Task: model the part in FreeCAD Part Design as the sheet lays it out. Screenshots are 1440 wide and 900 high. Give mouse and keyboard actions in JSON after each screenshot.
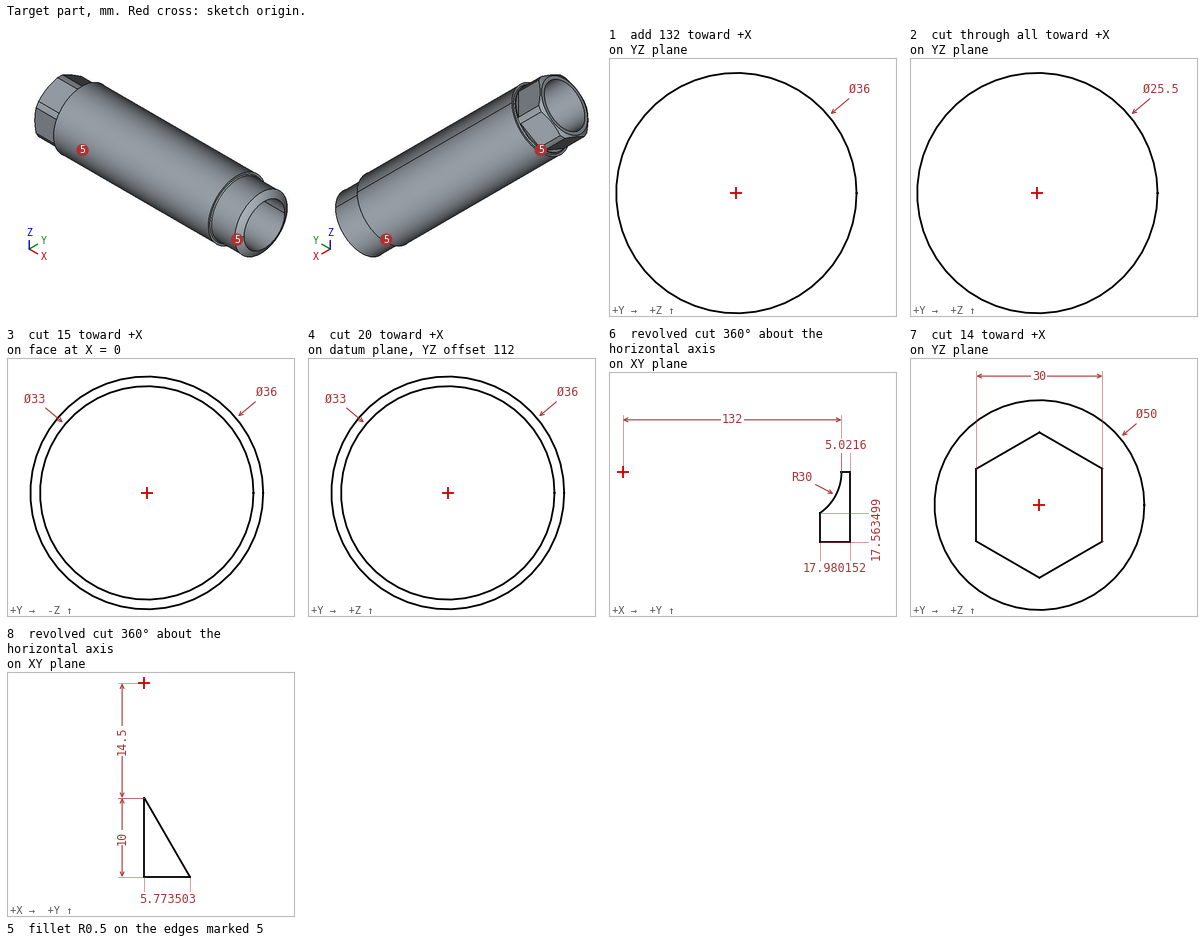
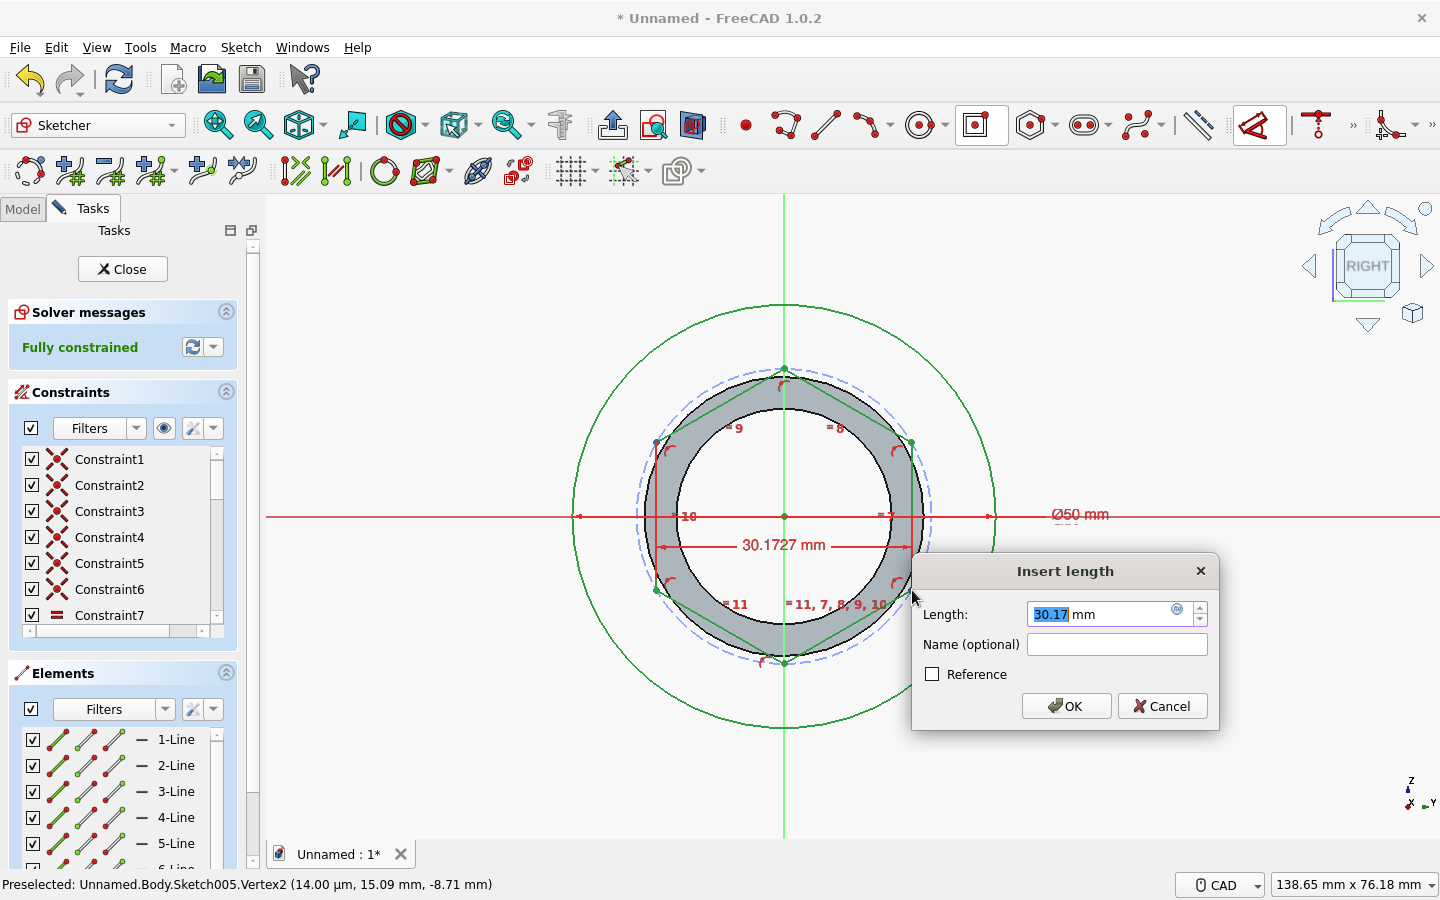
{"action": "type", "text": "30"}
{"action": "key", "text": "Return"}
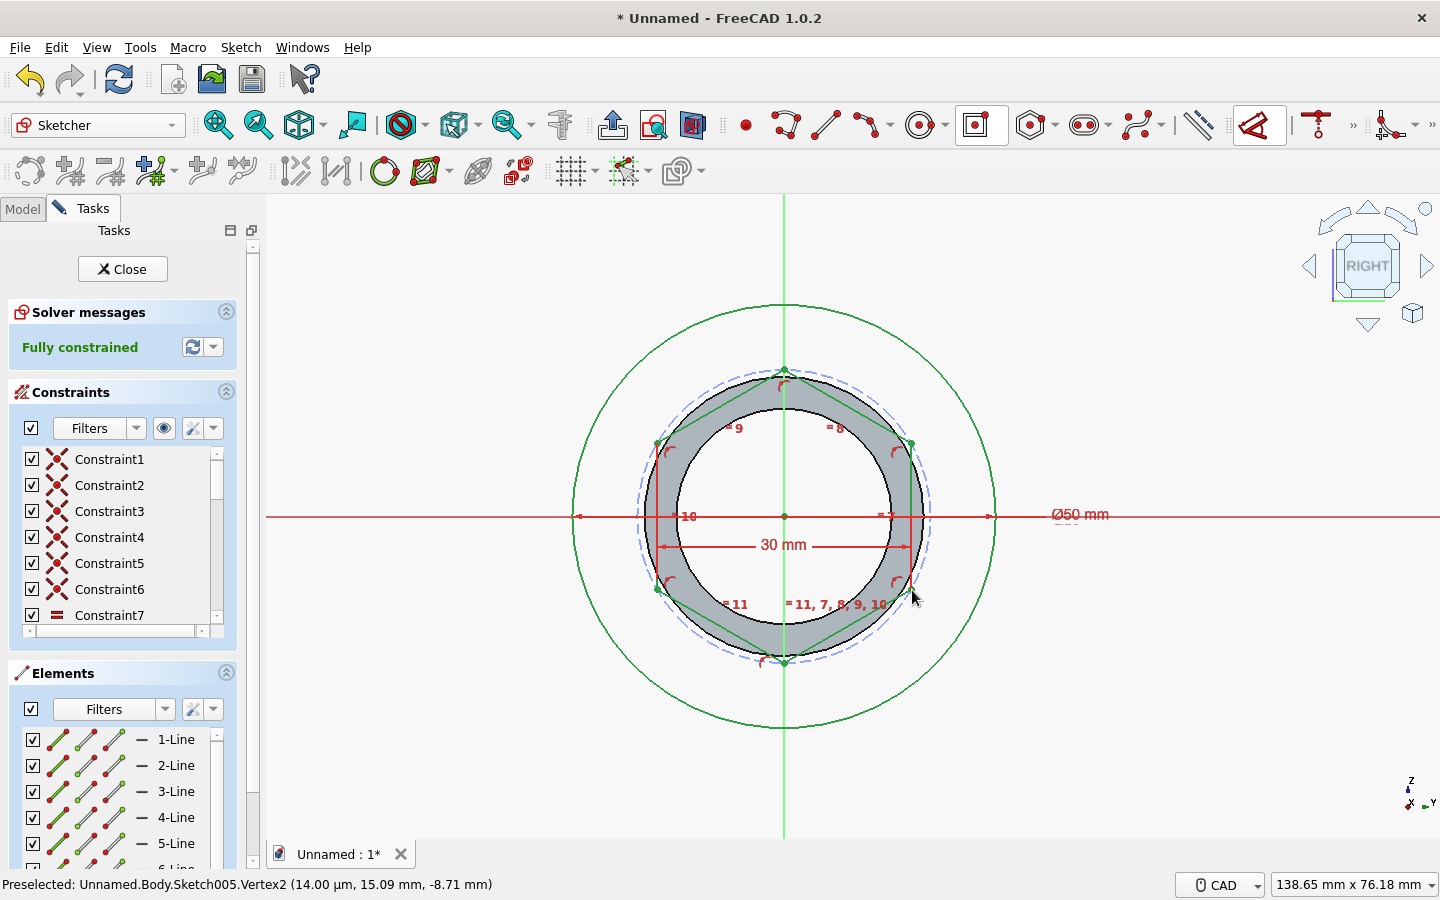
{"action": "left_click", "coordinate": [123, 269]}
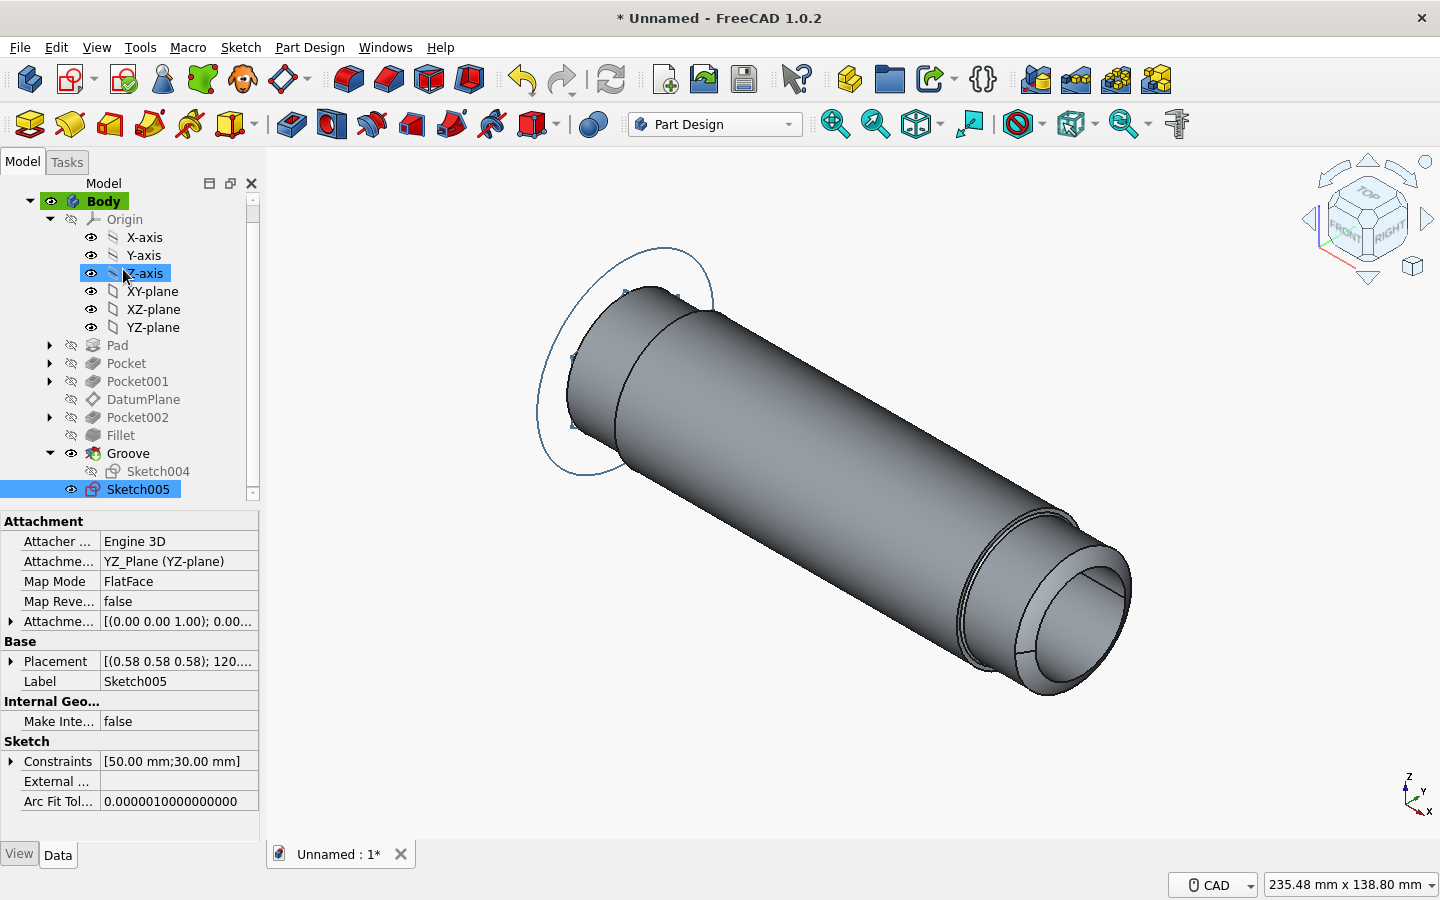
{"action": "left_click", "coordinate": [292, 124]}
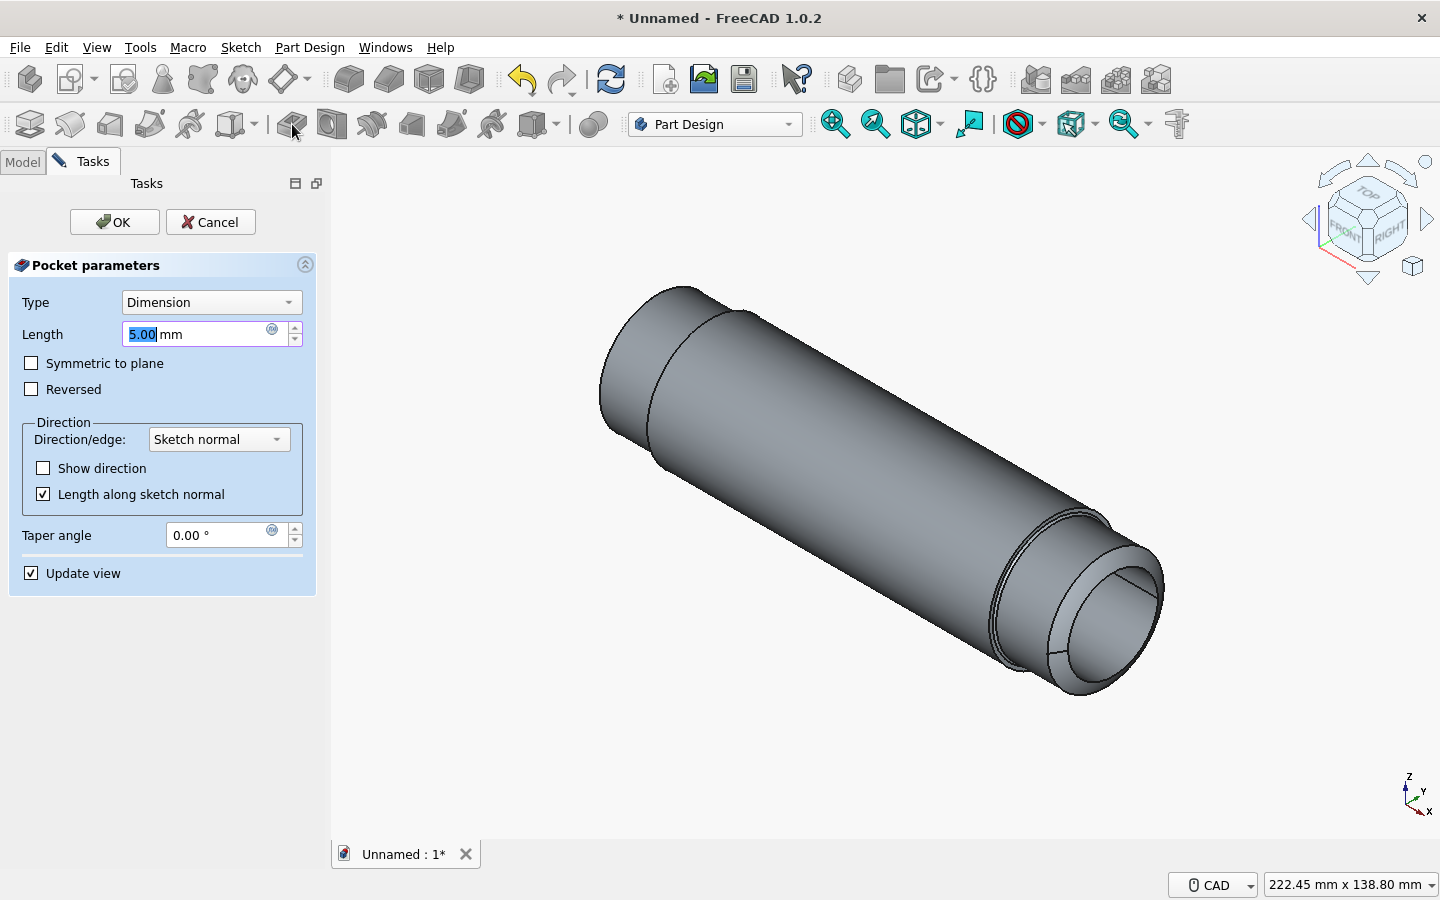
{"action": "type", "text": "14"}
{"action": "key", "text": "Tab"}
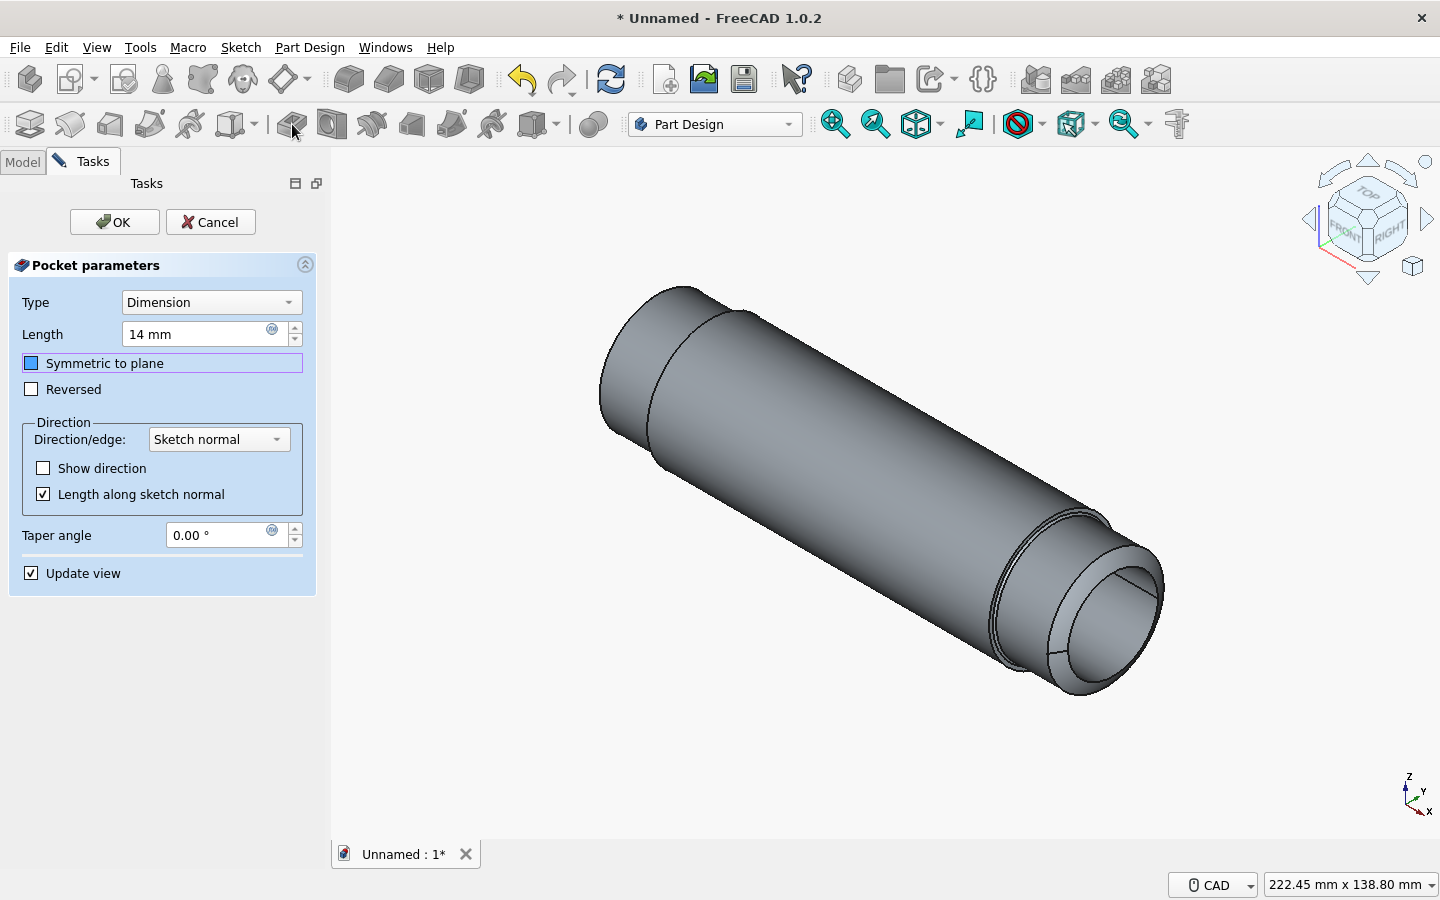
{"action": "left_click", "coordinate": [30, 389]}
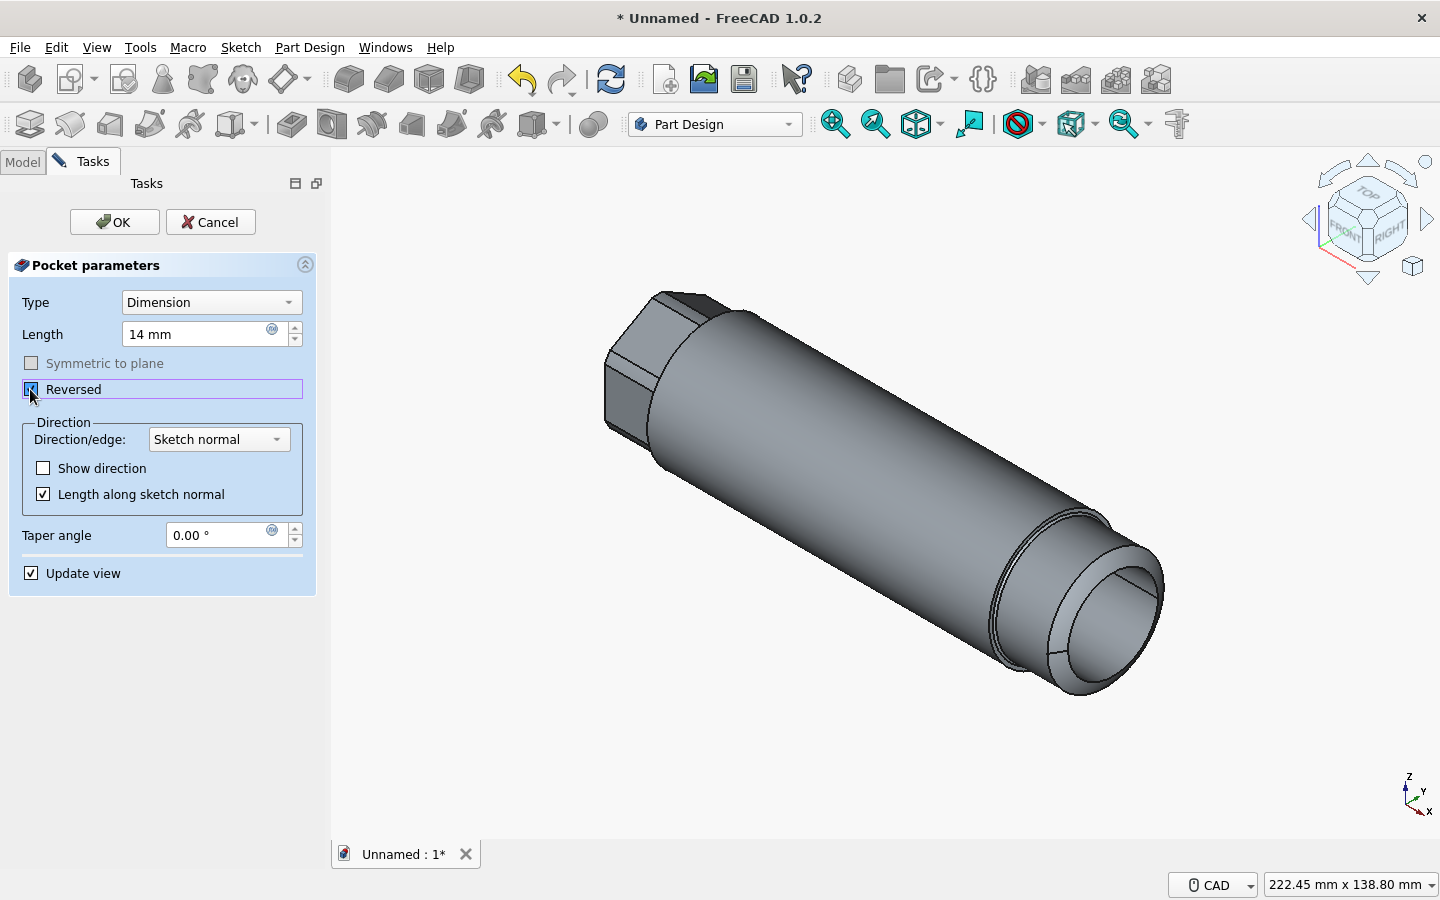
{"action": "left_click", "coordinate": [115, 222]}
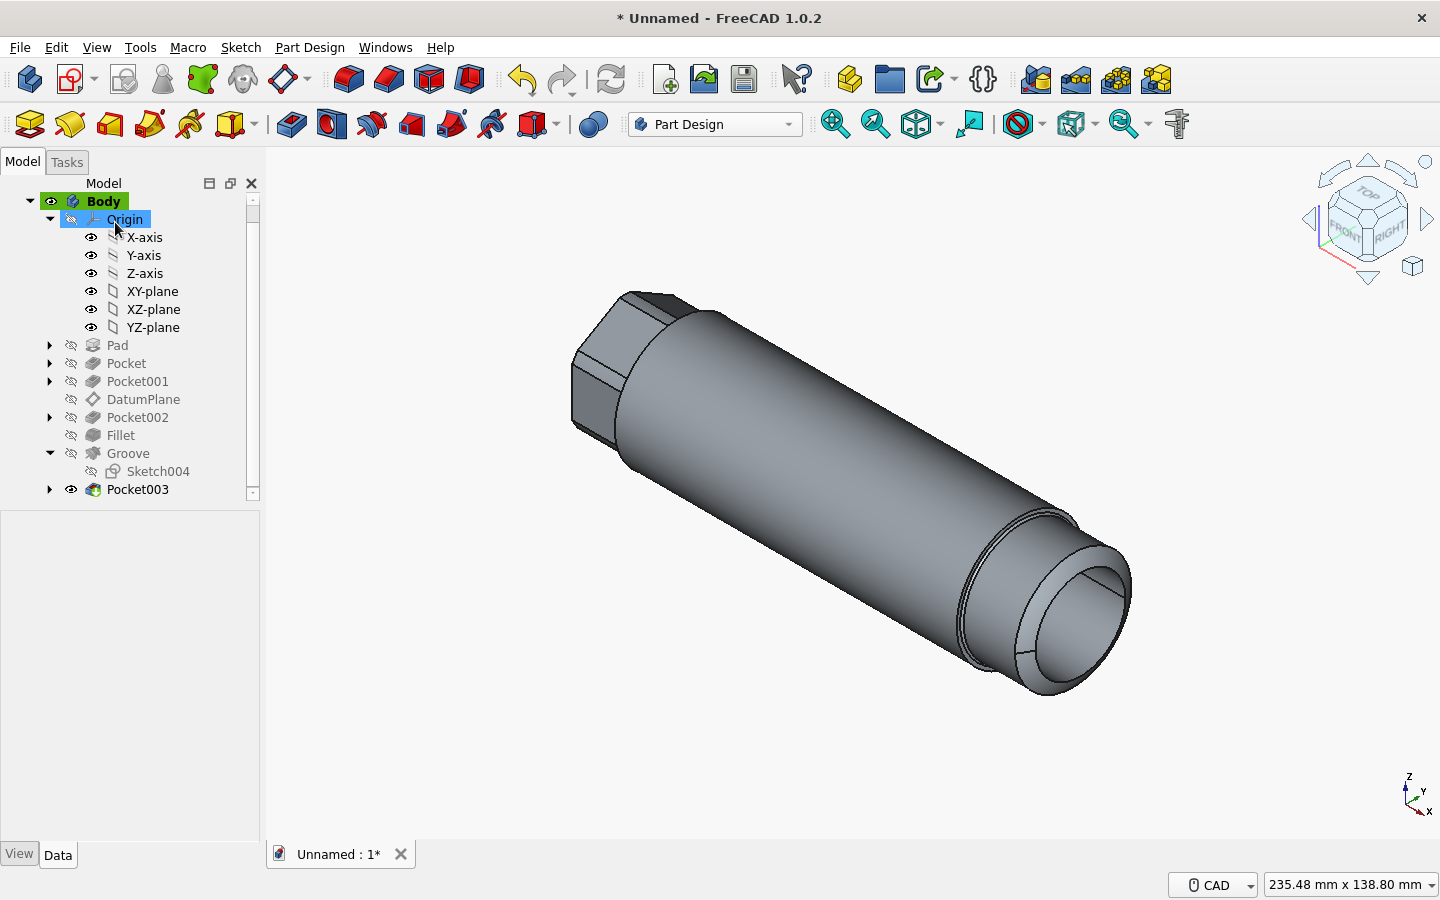
{"action": "left_click", "coordinate": [70, 80]}